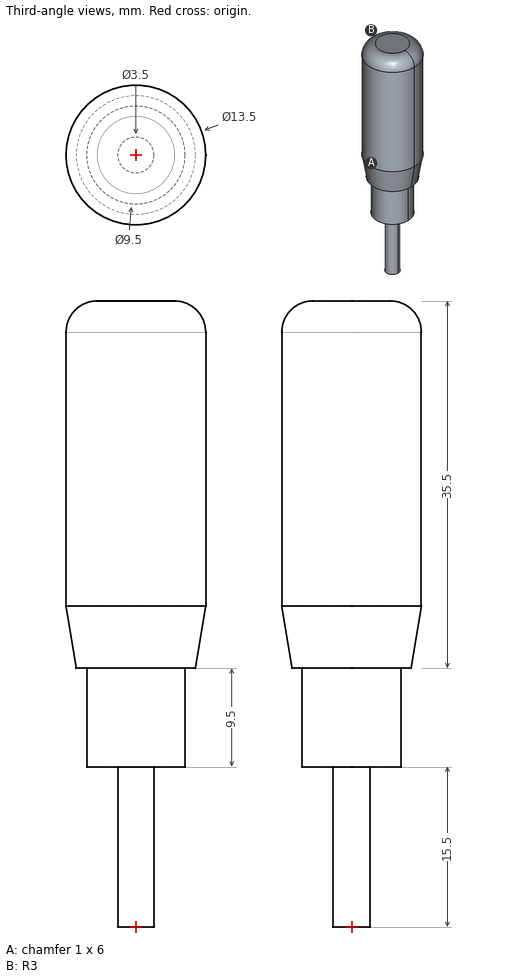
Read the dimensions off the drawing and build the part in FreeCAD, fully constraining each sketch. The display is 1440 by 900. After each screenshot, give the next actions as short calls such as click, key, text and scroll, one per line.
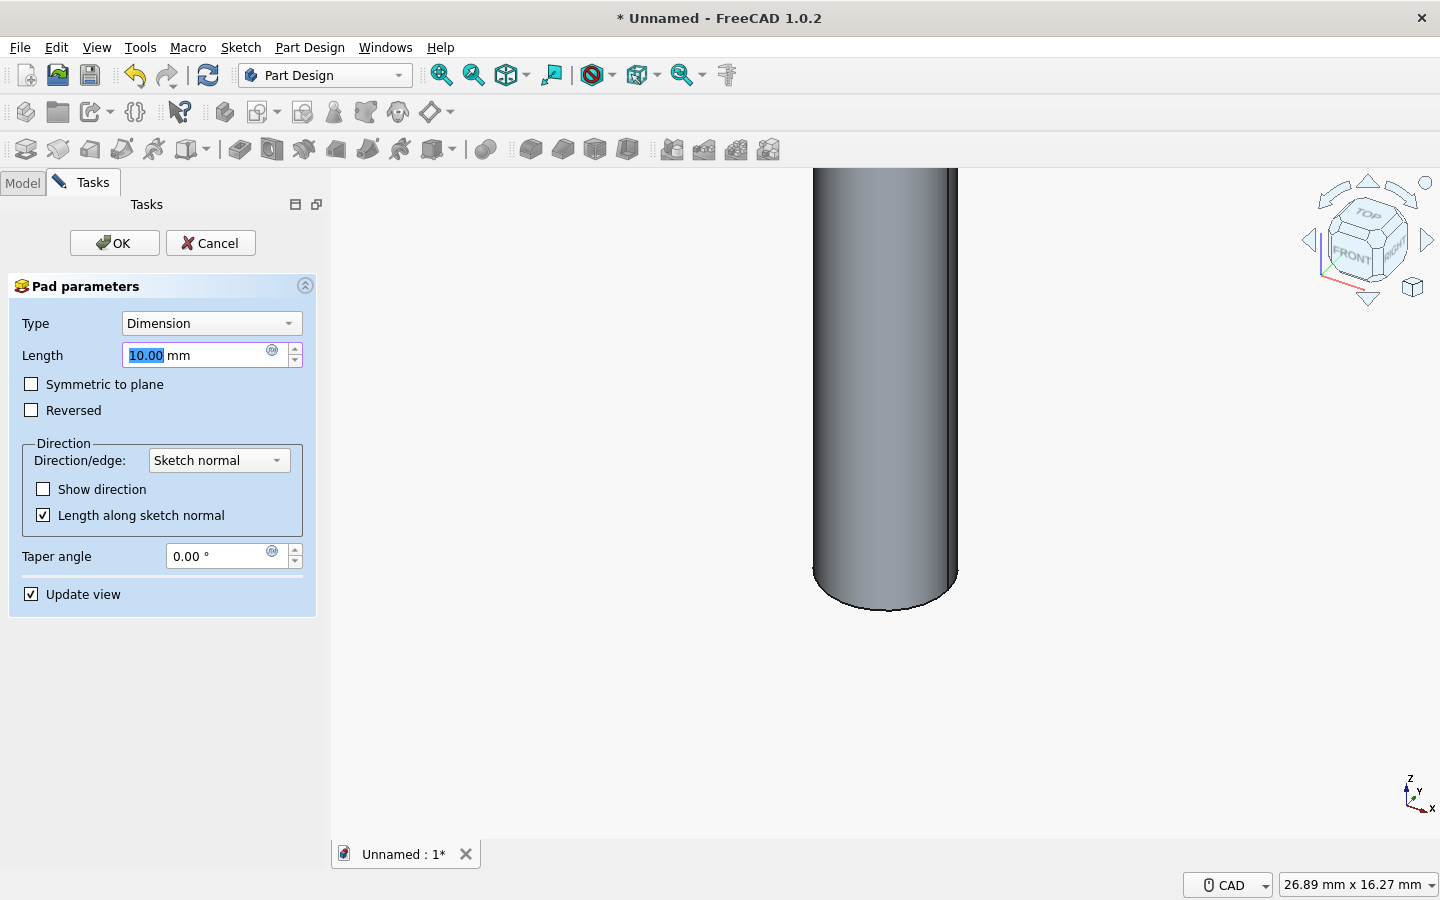
text(9.5)
key(Tab)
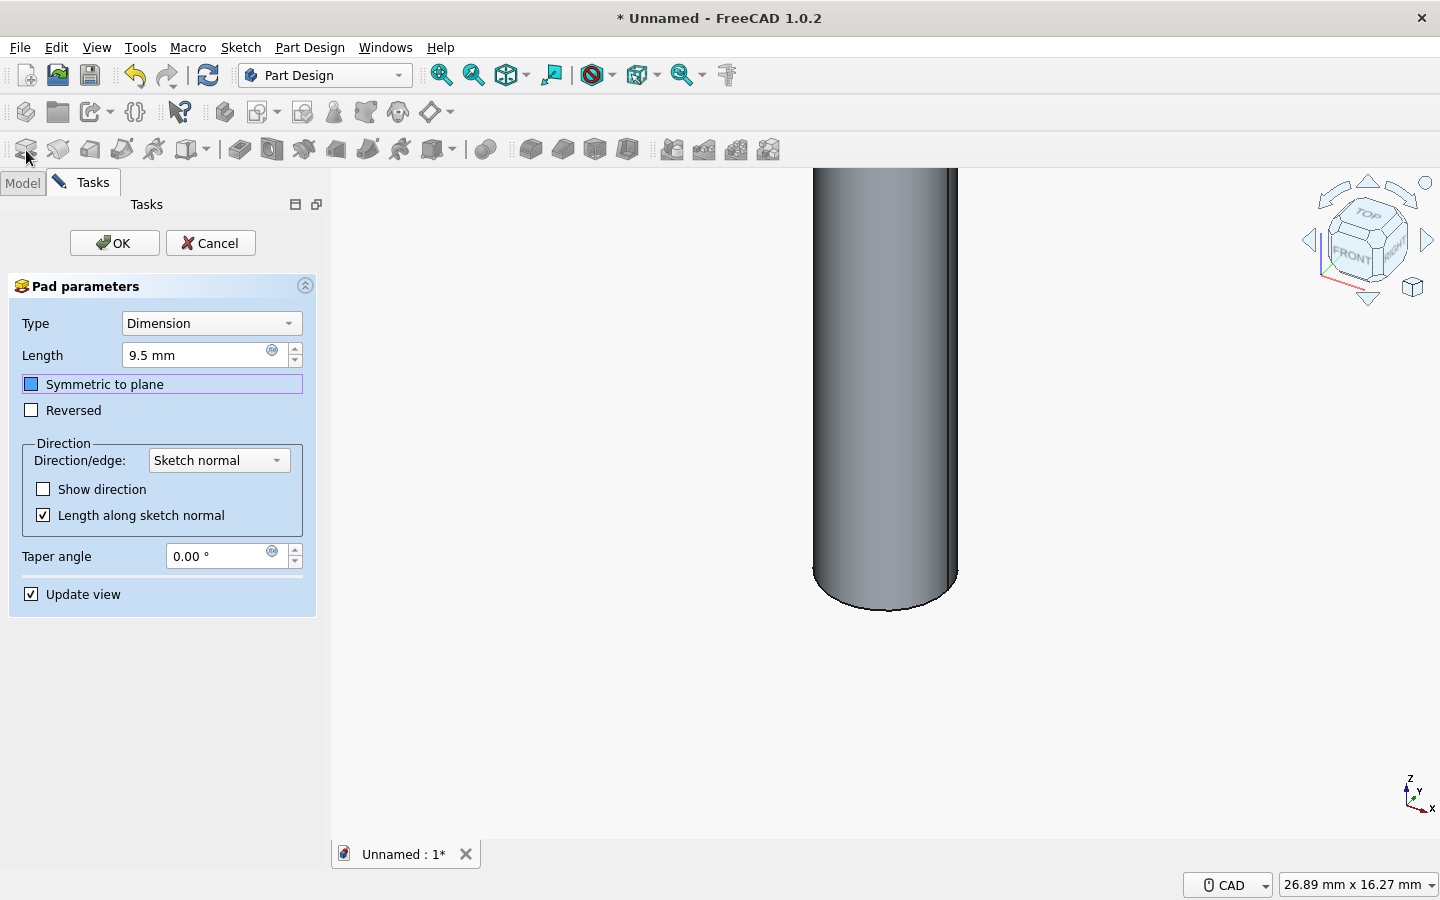
click(115, 243)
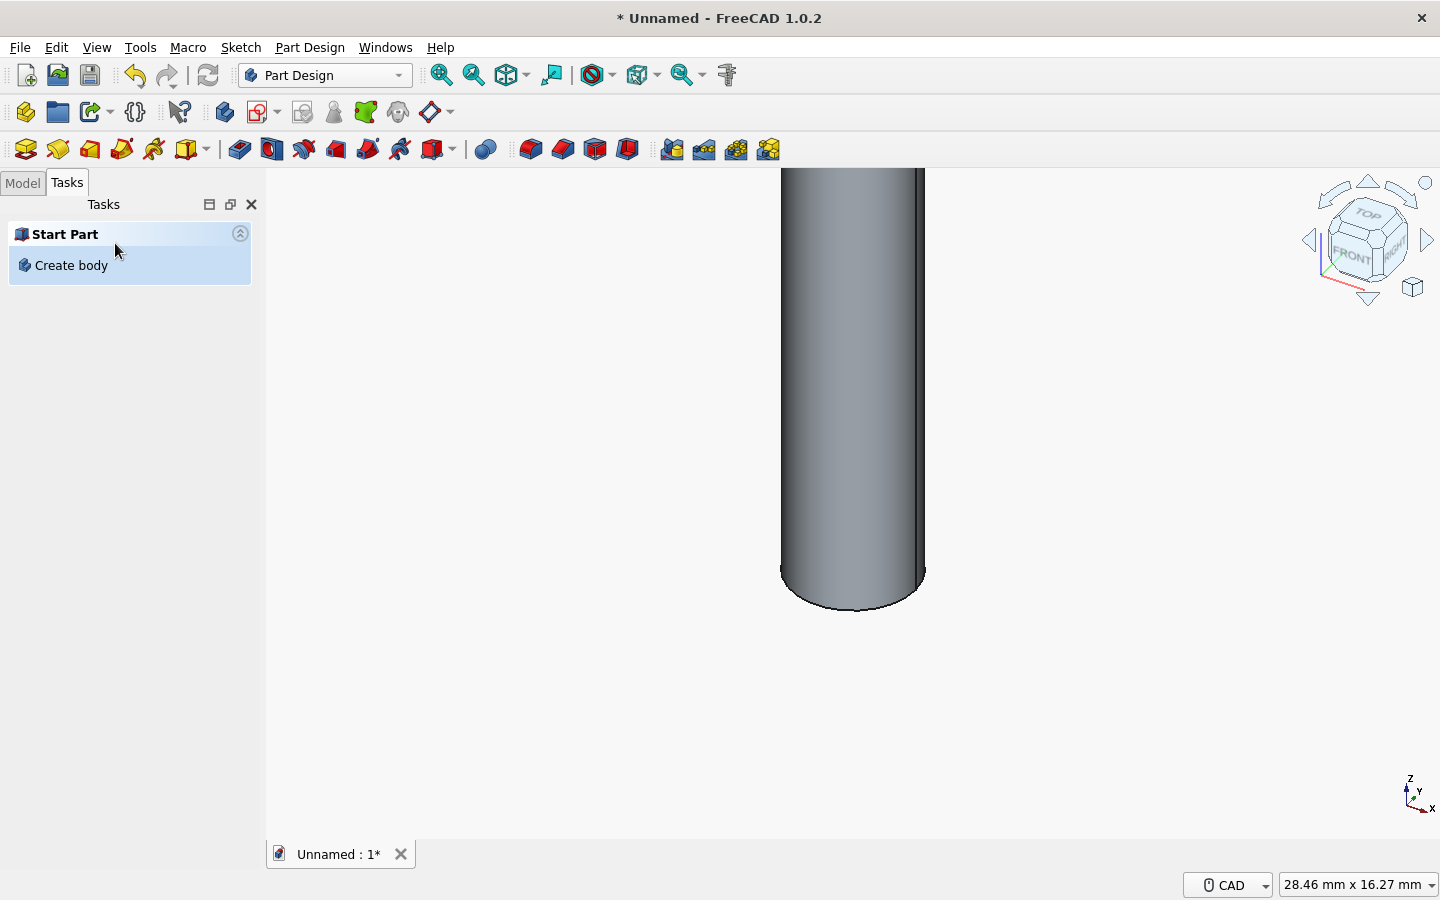
click(442, 76)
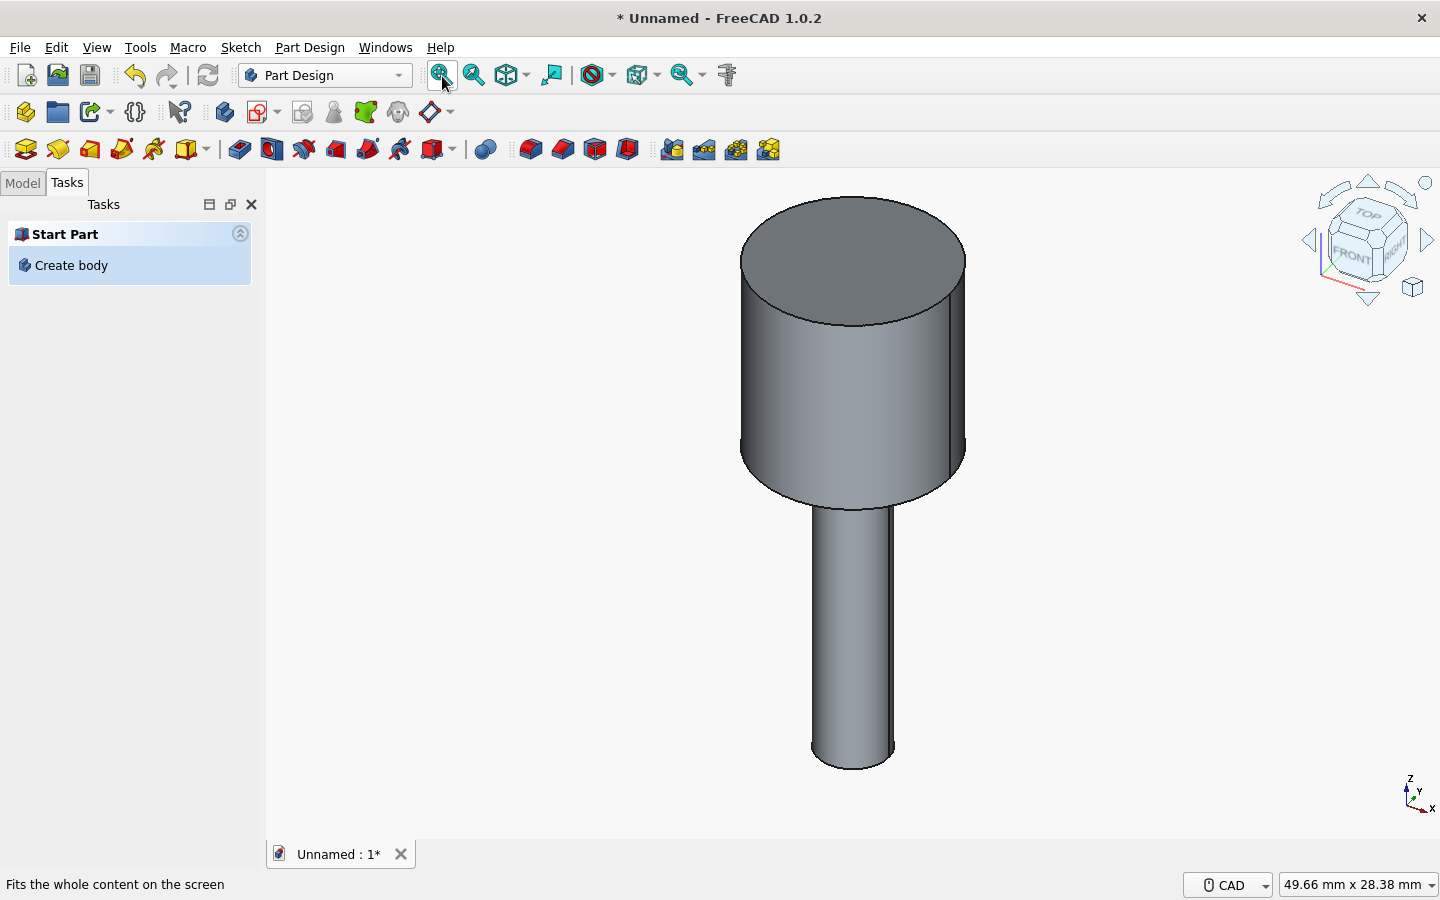
click(853, 260)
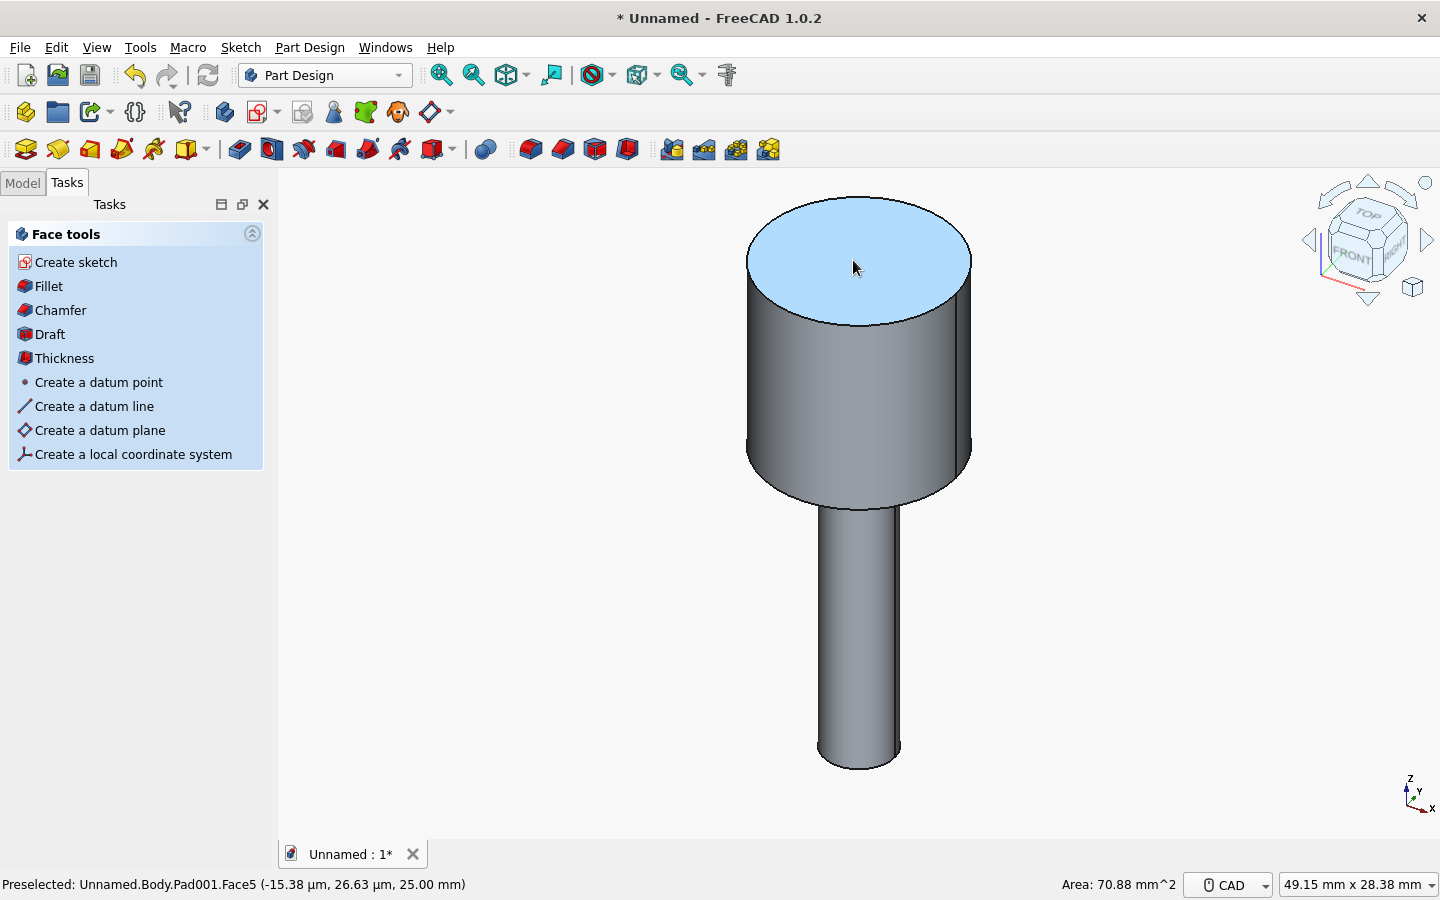
click(258, 112)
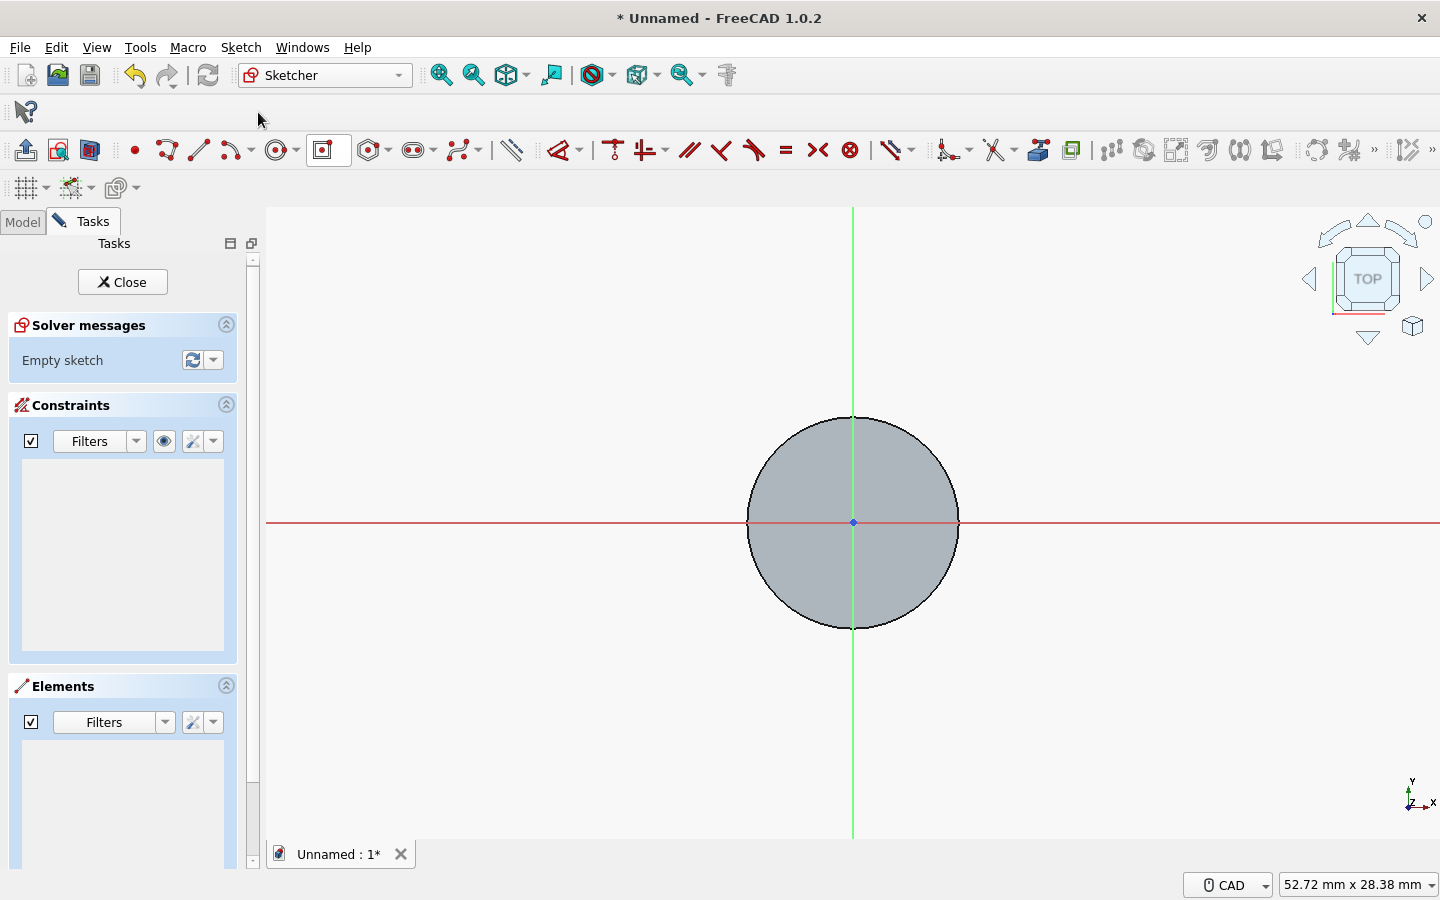
scroll(992, 523, up, 2)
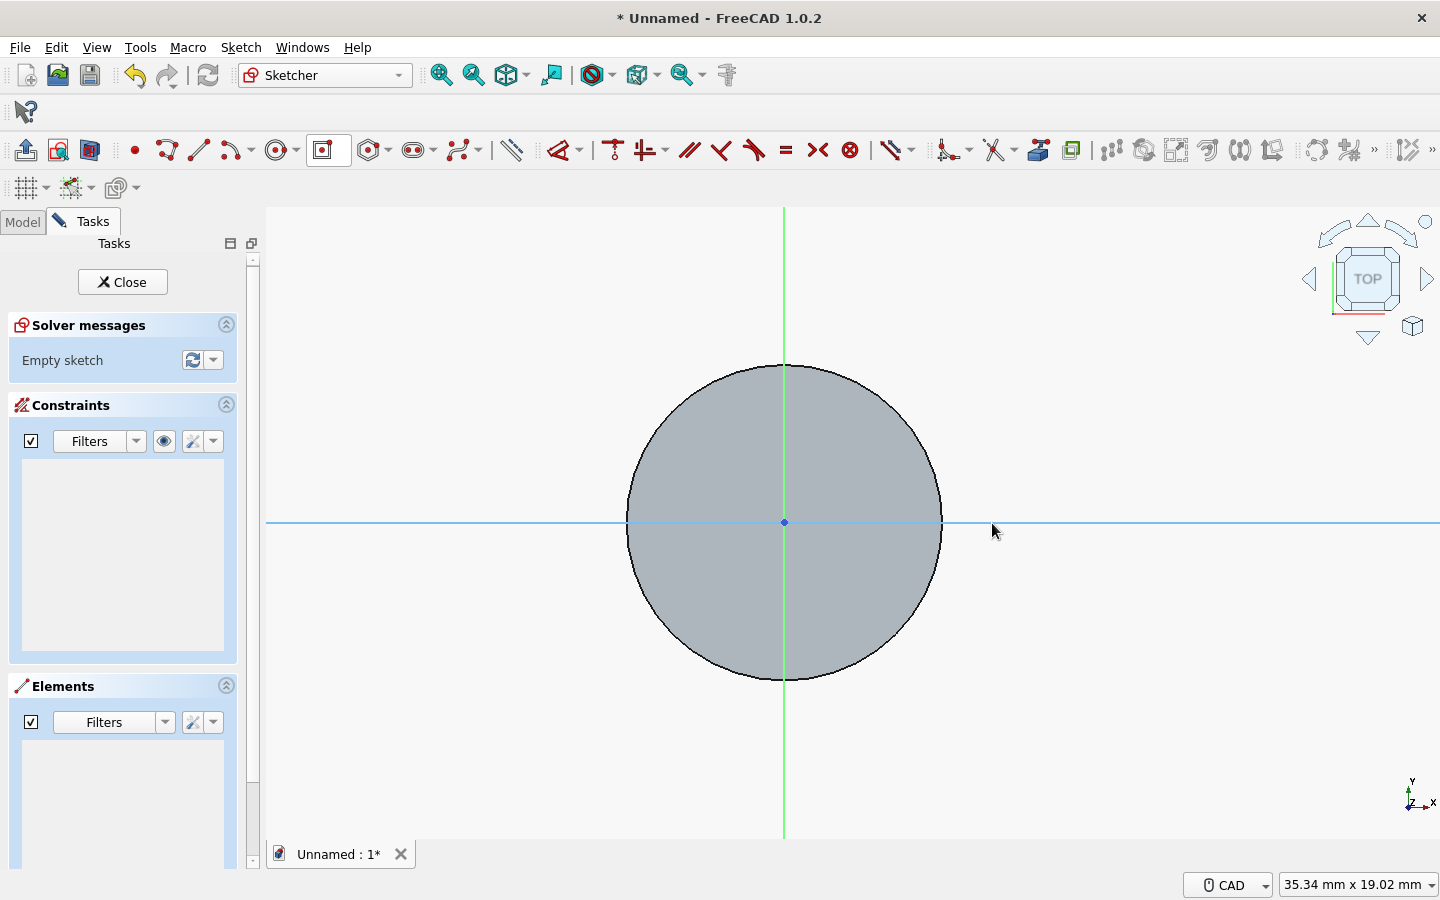
click(276, 150)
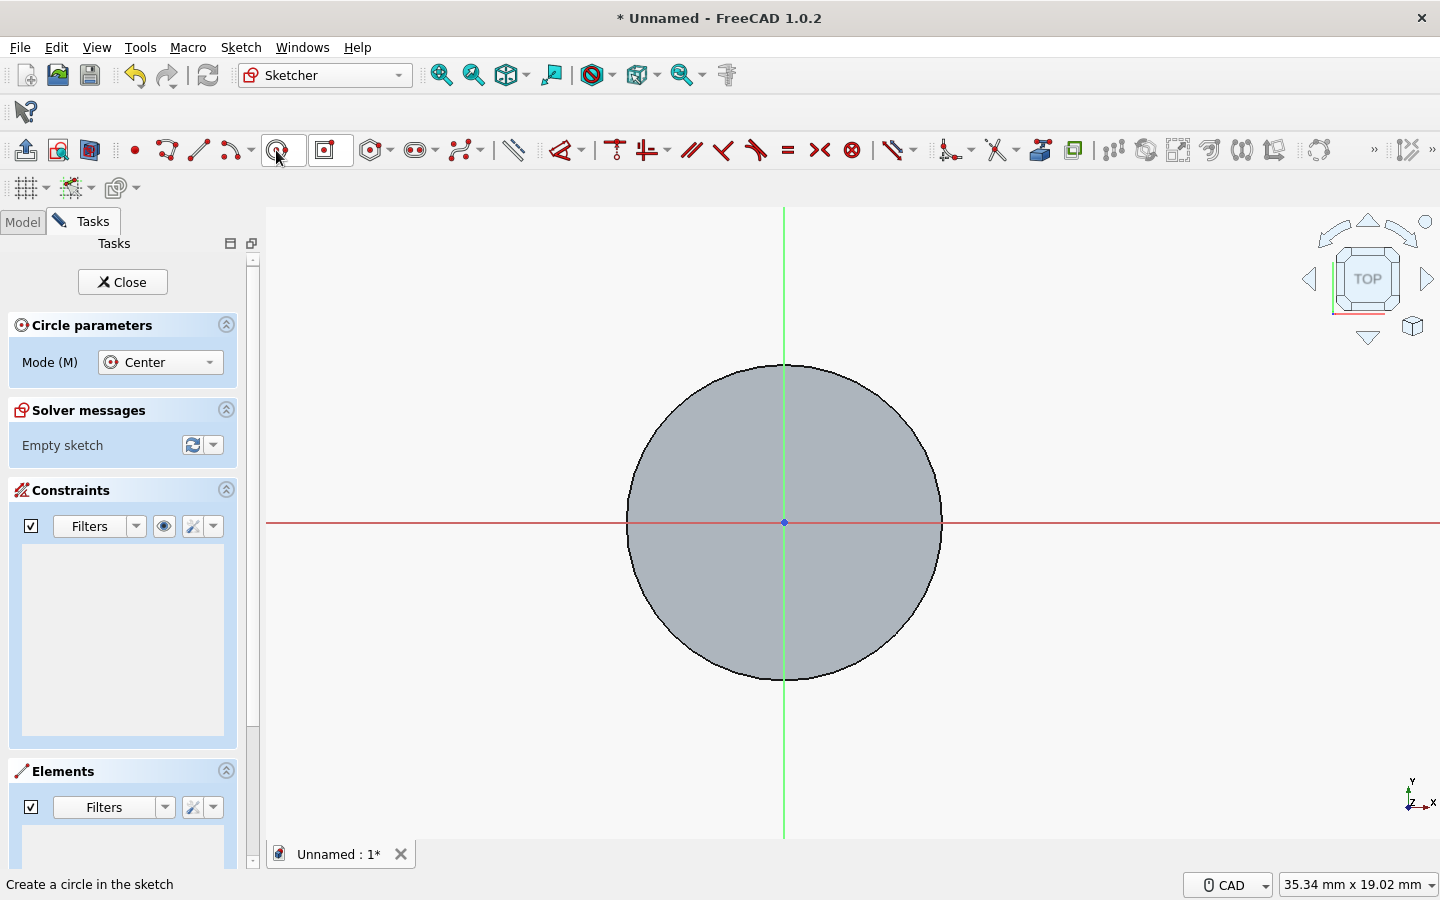
click(784, 523)
click(943, 364)
key(Escape)